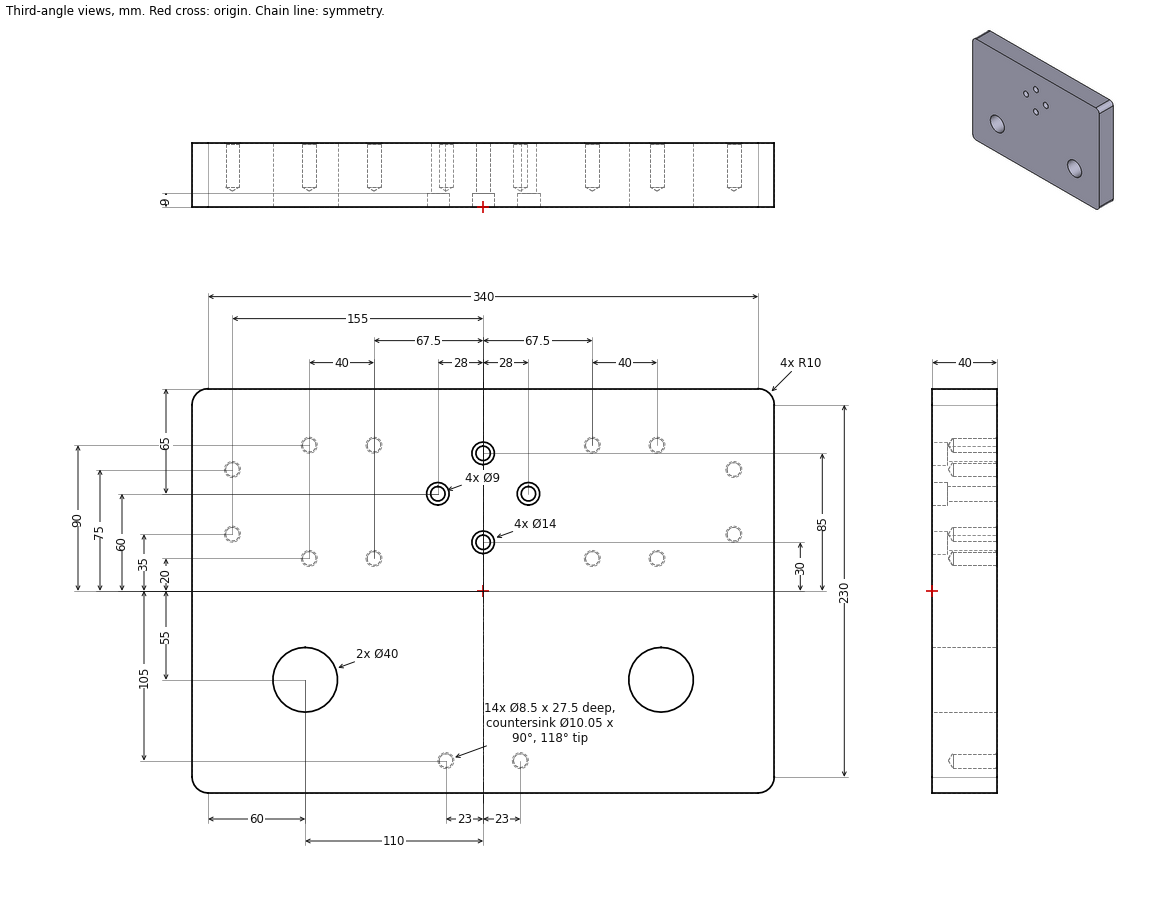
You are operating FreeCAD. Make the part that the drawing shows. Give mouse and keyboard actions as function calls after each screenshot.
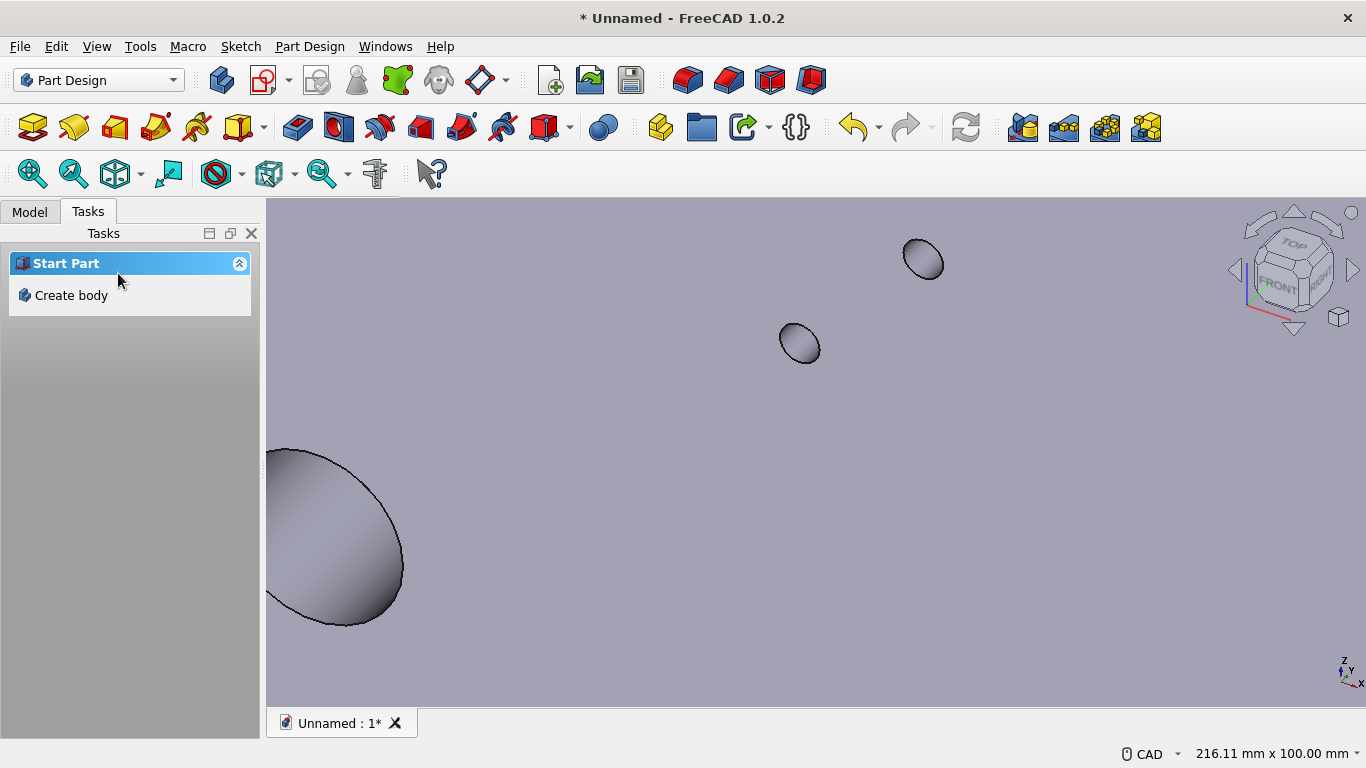
click(33, 174)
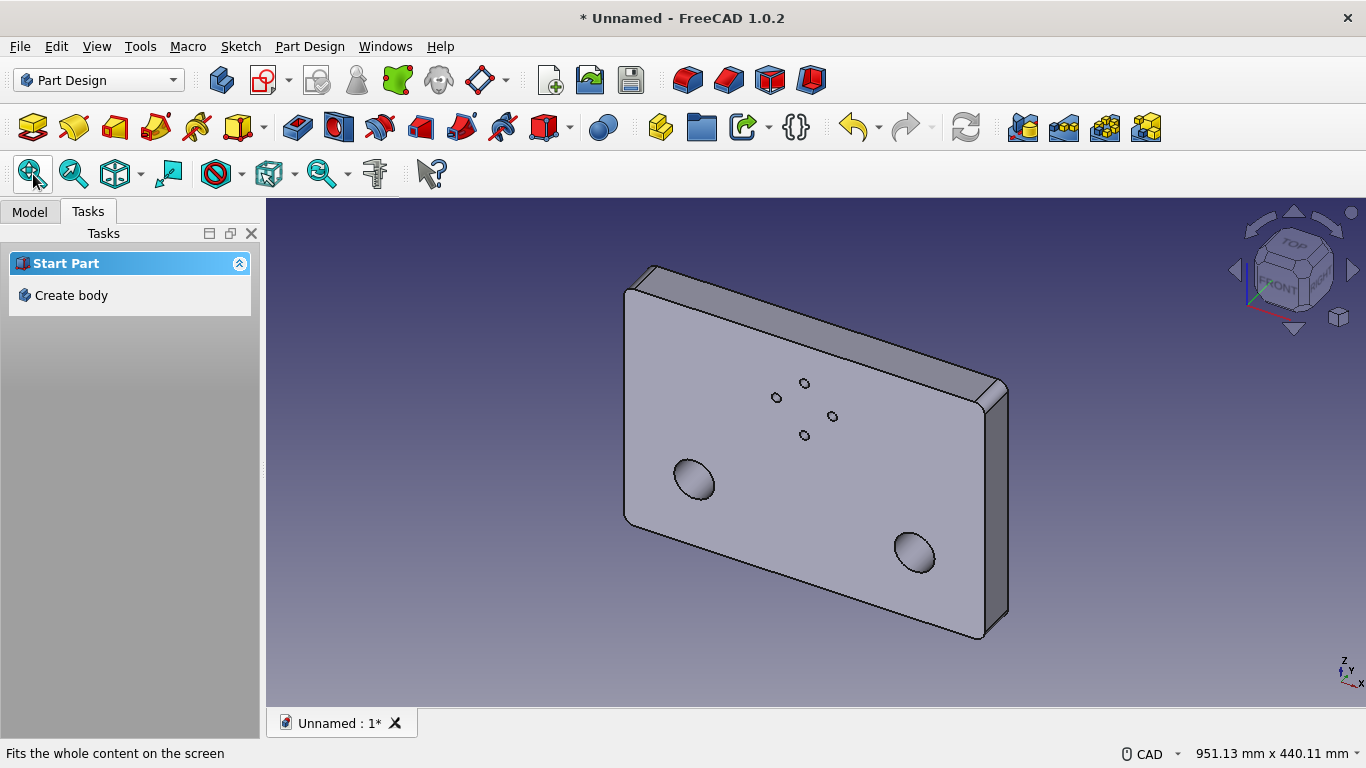
click(701, 395)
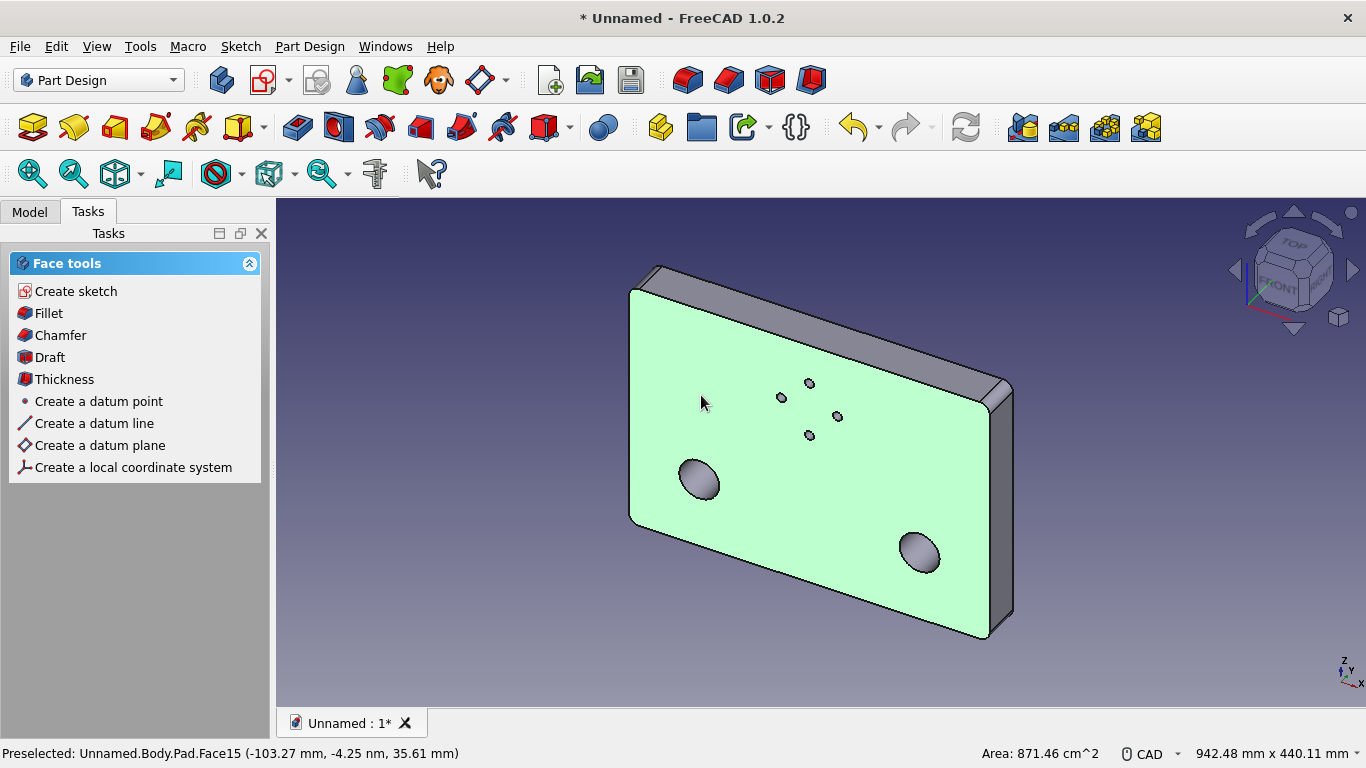
click(262, 80)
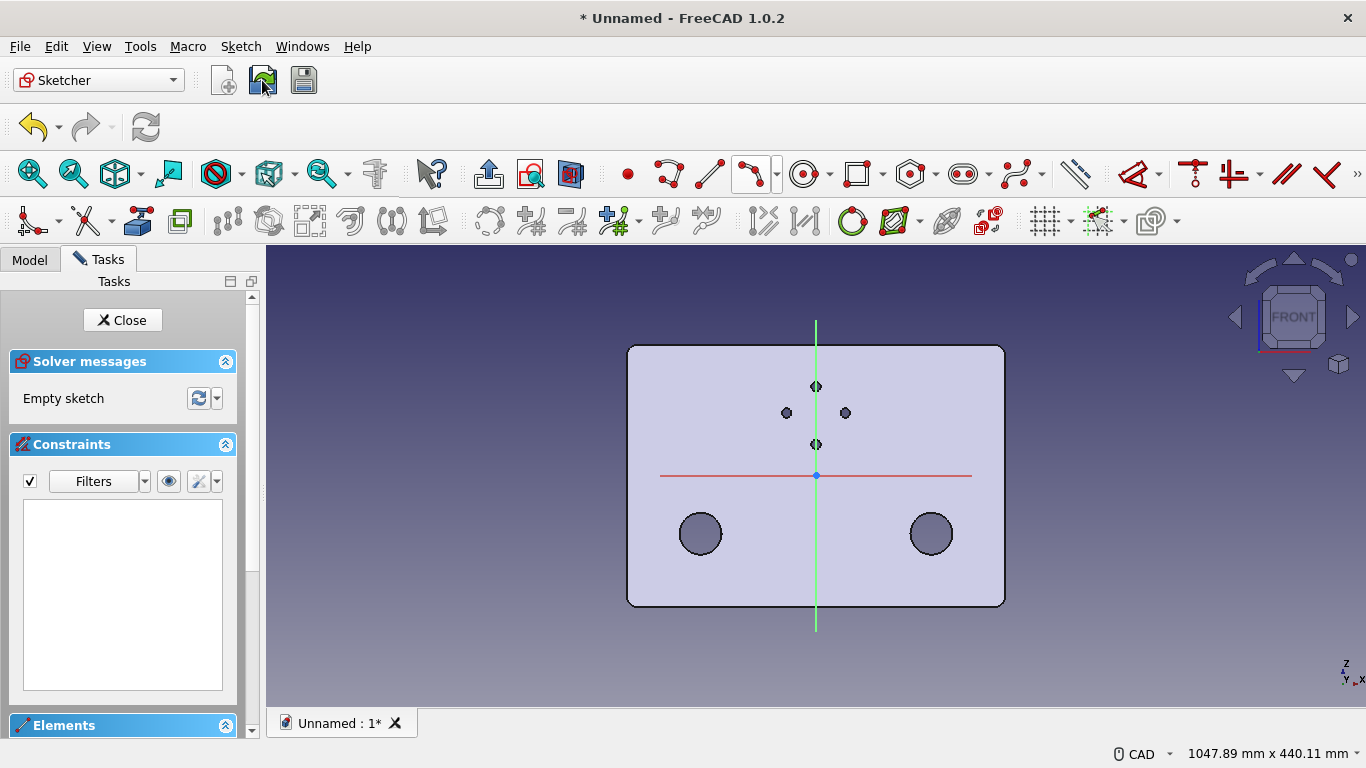
scroll(856, 400, up, 5)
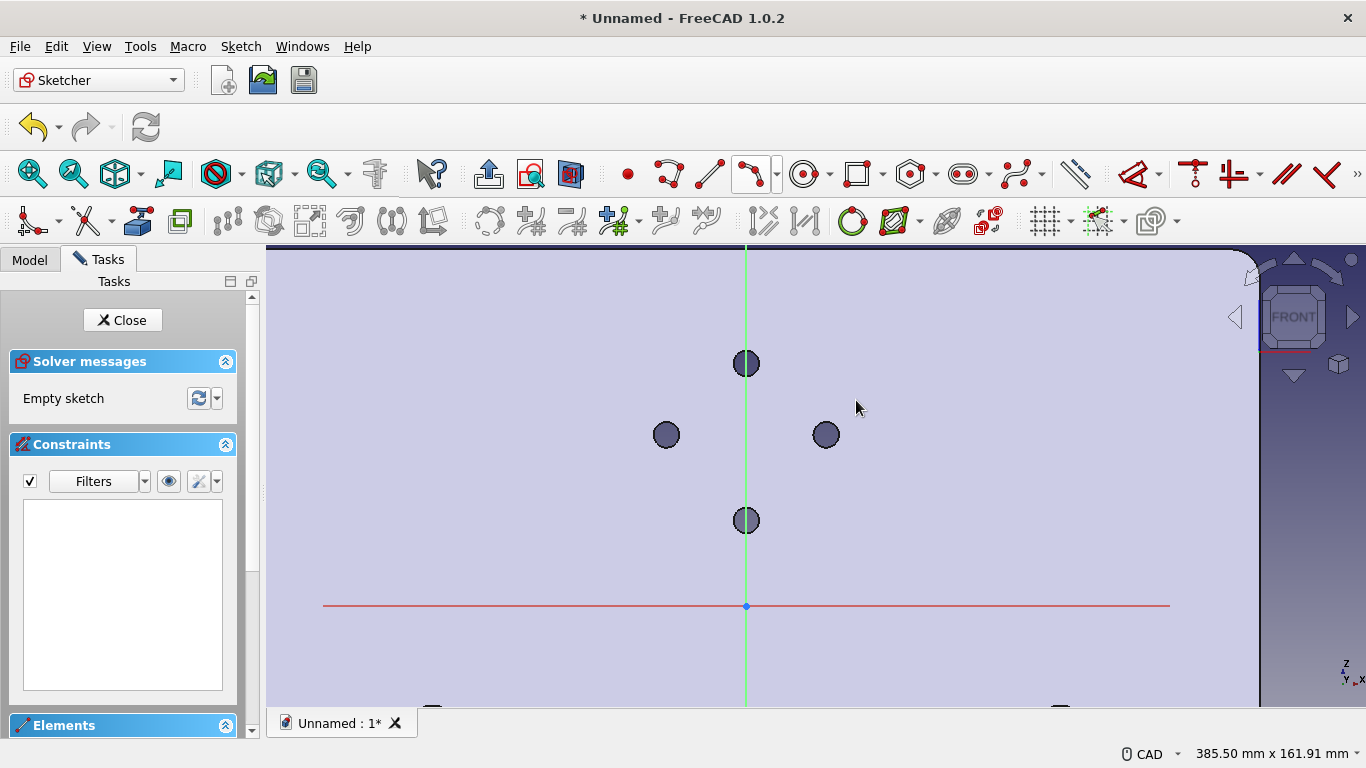
click(804, 174)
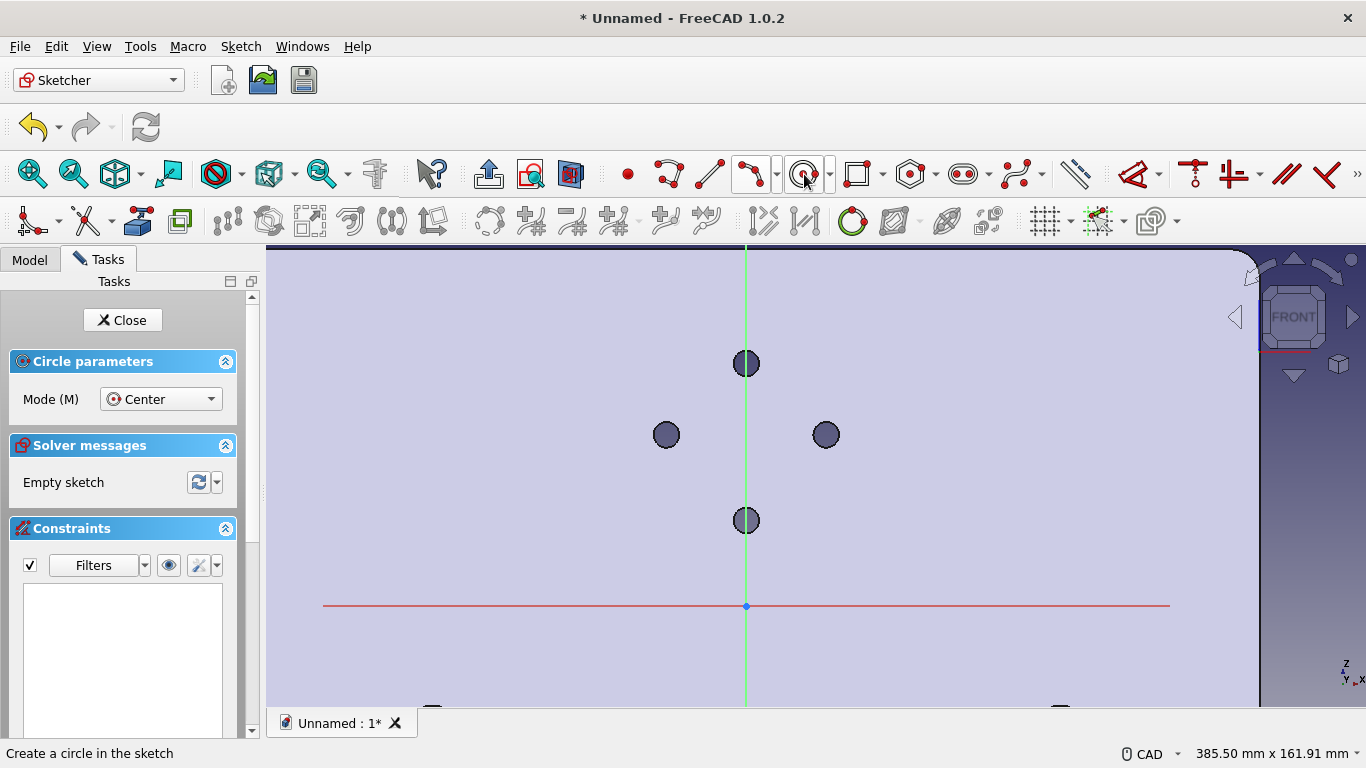
click(746, 520)
move(760, 506)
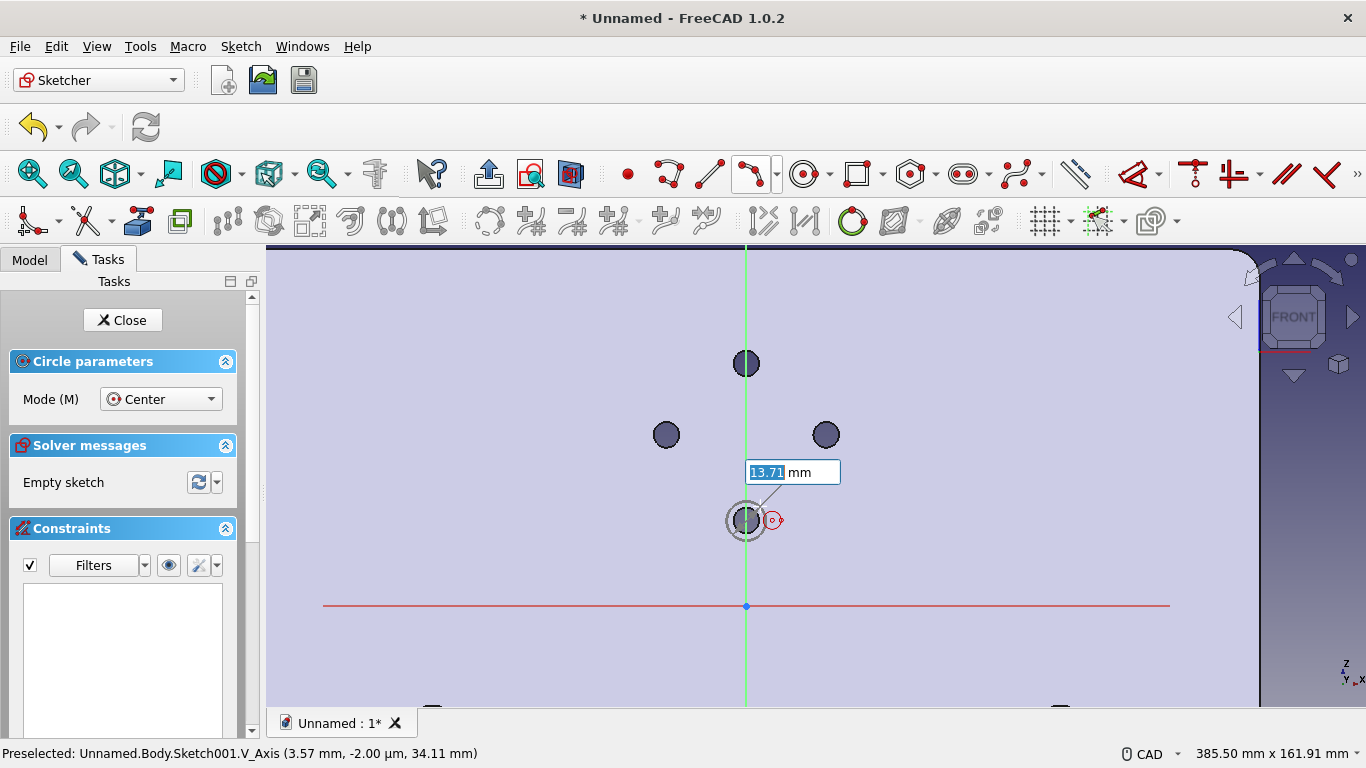
text(14)
key(Return)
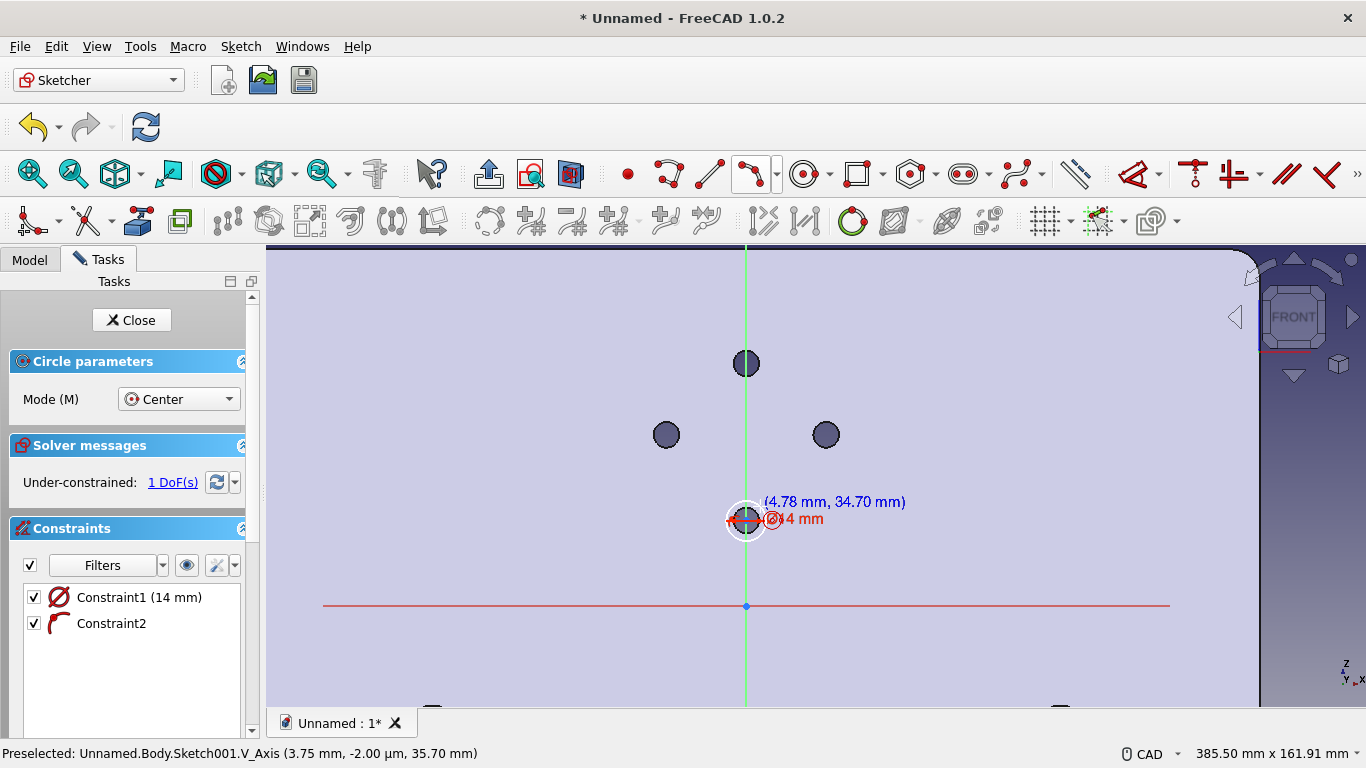
click(666, 435)
move(681, 421)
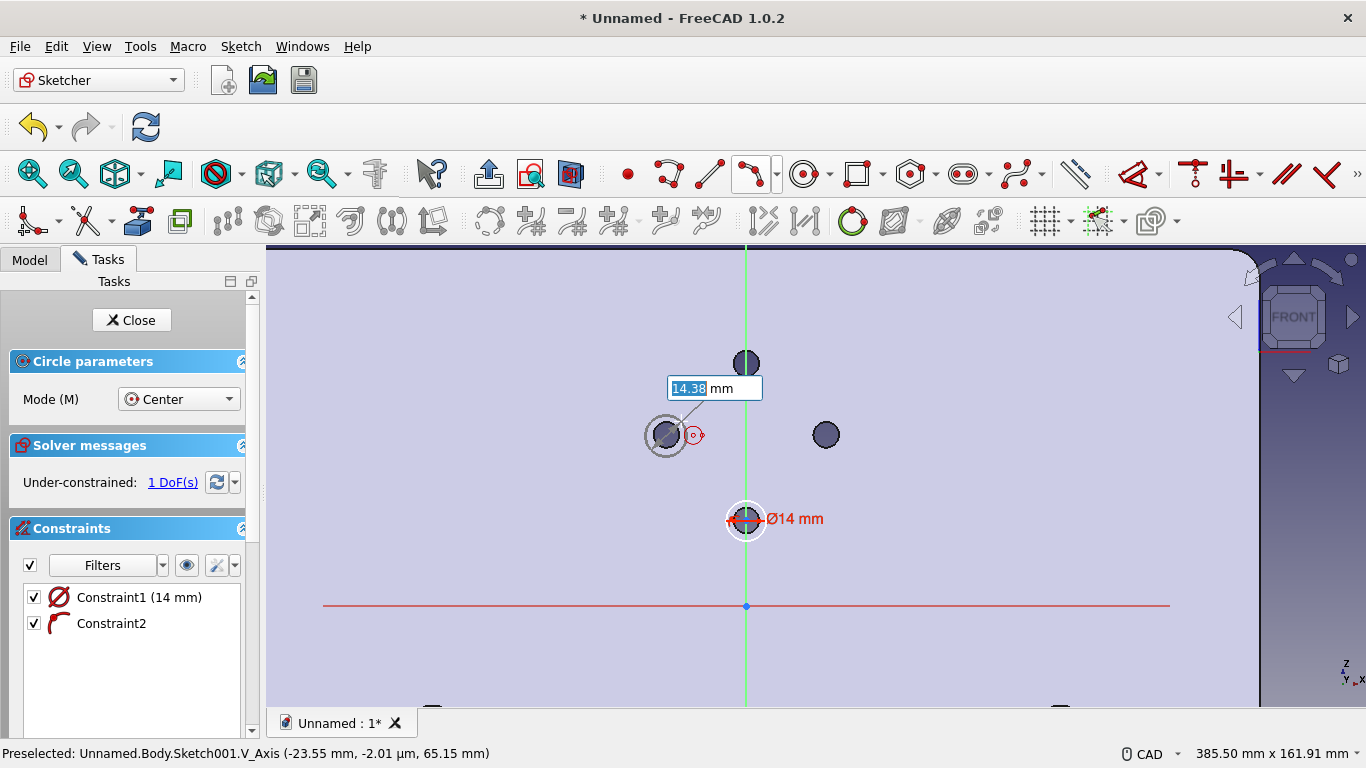
text(14)
key(Return)